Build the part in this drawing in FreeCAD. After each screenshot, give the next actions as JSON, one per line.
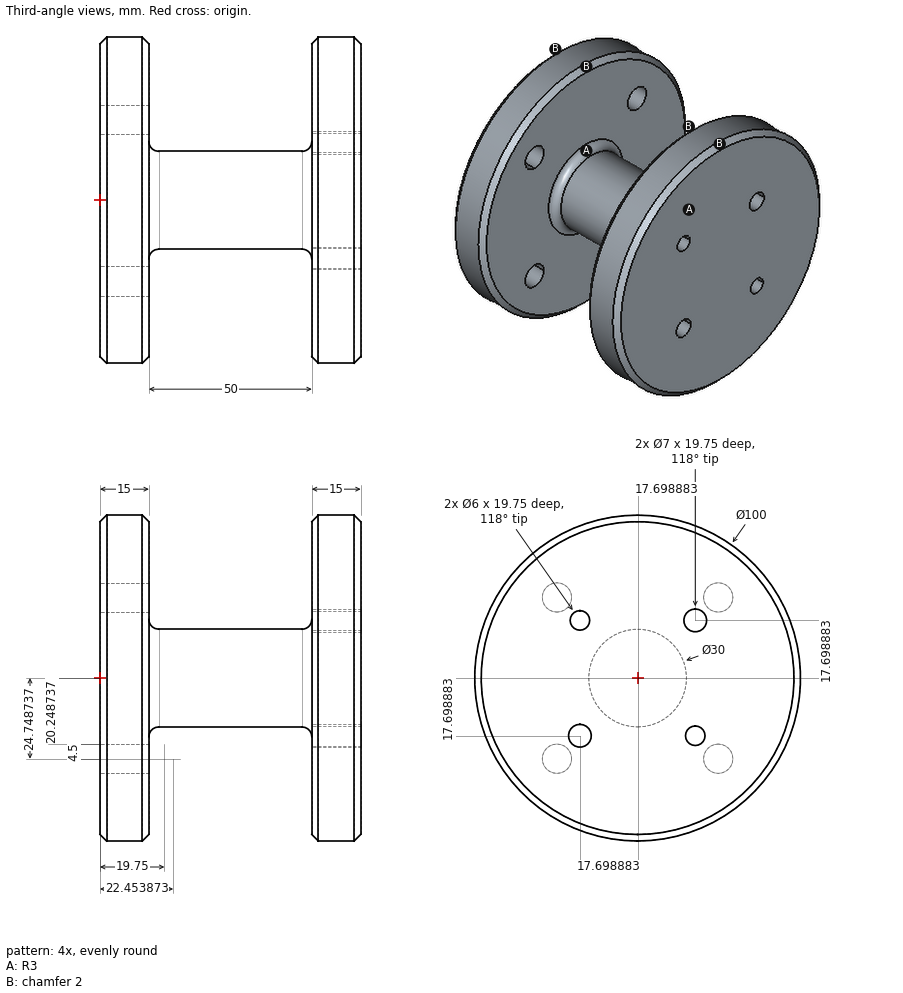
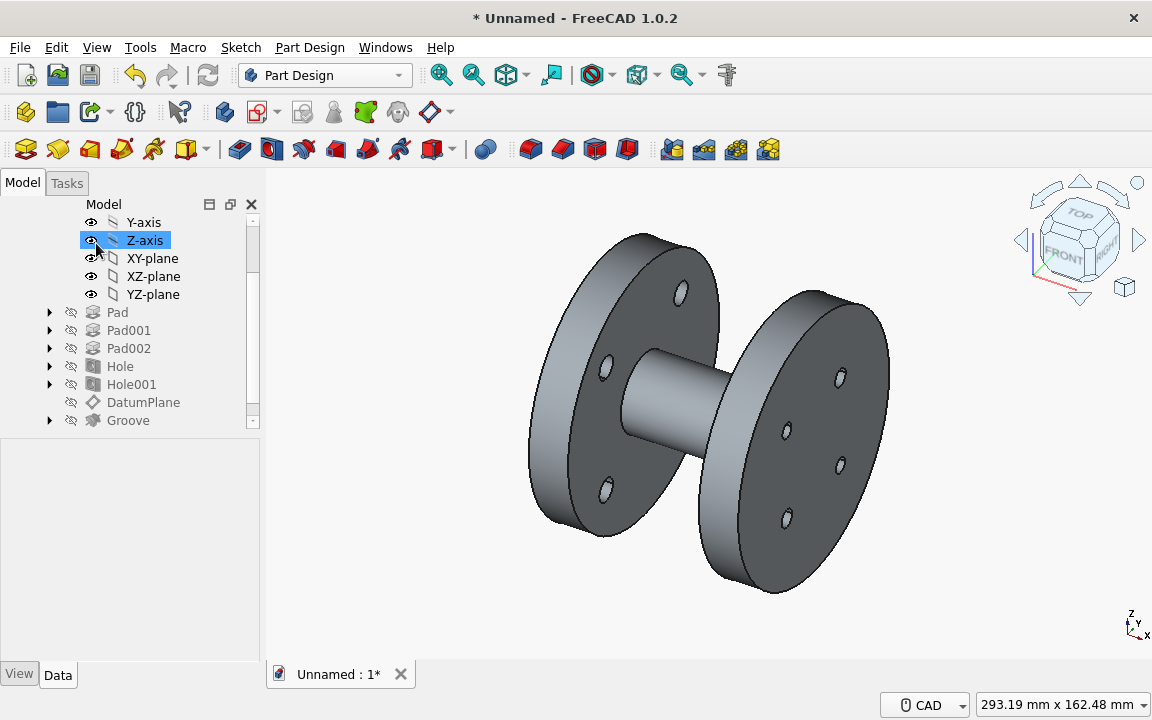
{"action": "key", "text": "0"}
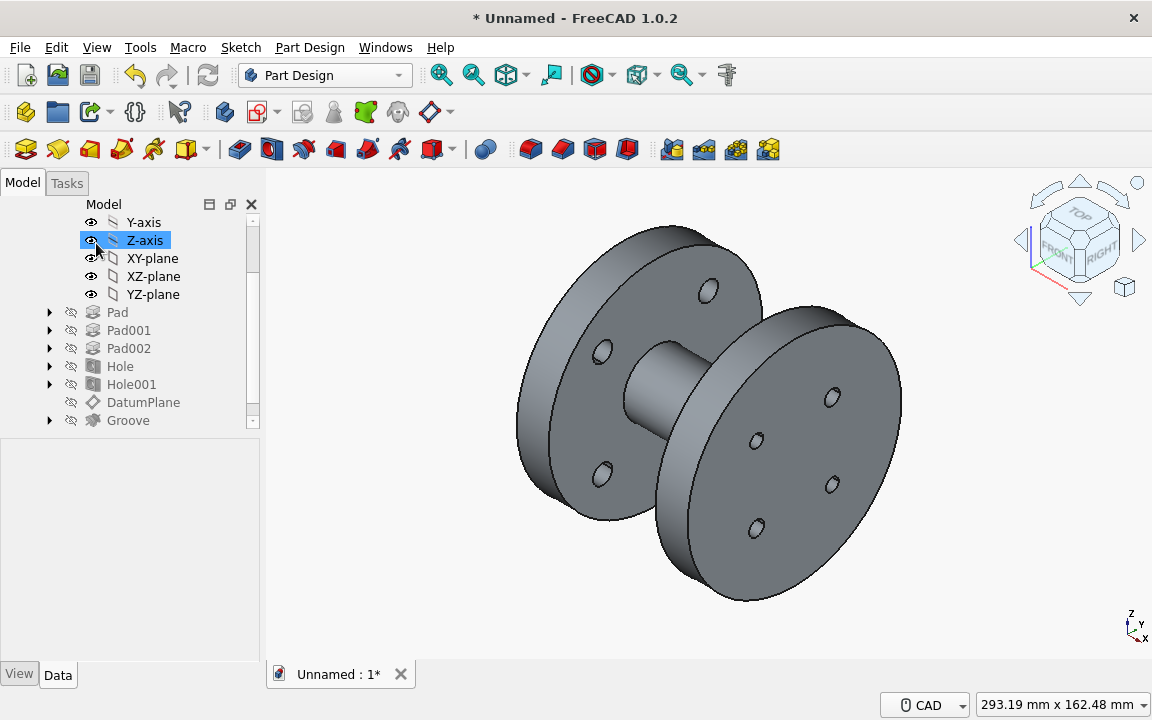
{"action": "key", "text": "2"}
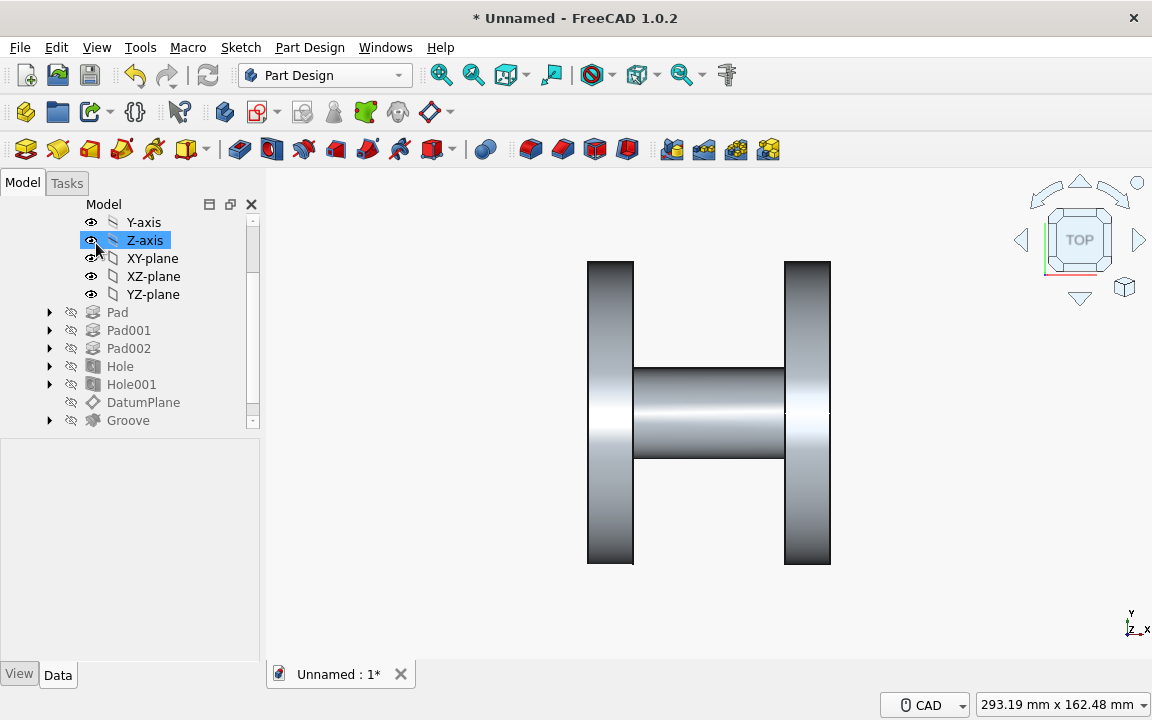
{"action": "key", "text": "1"}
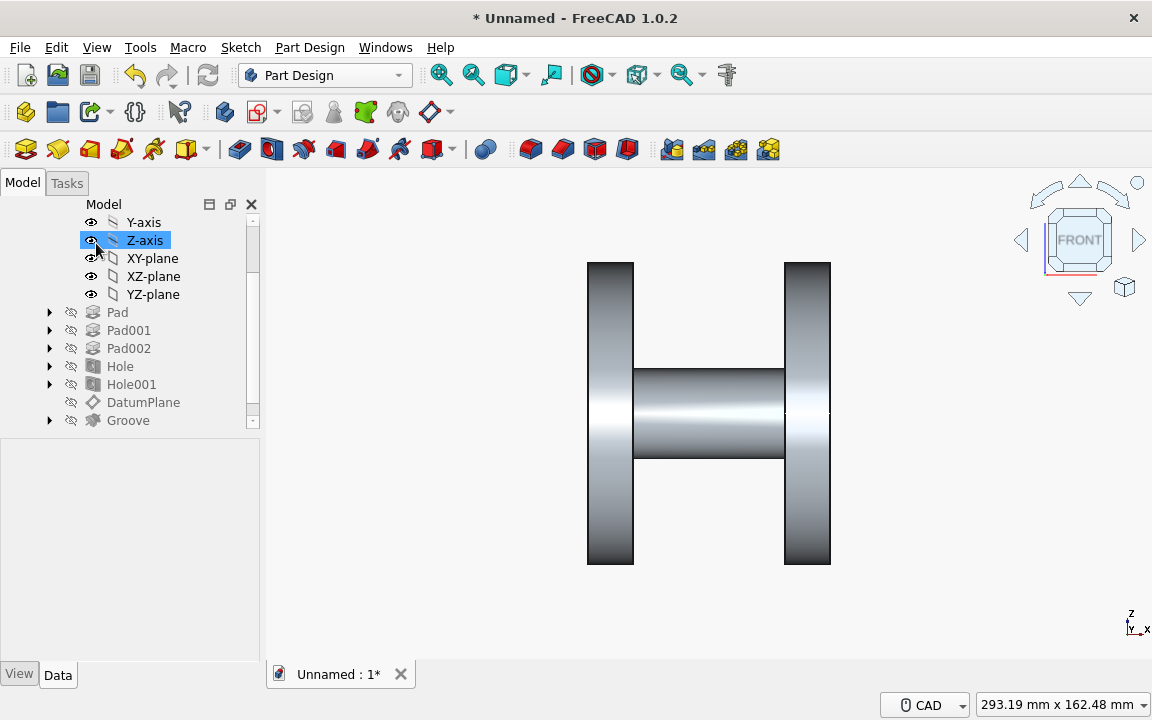
{"action": "key", "text": "3"}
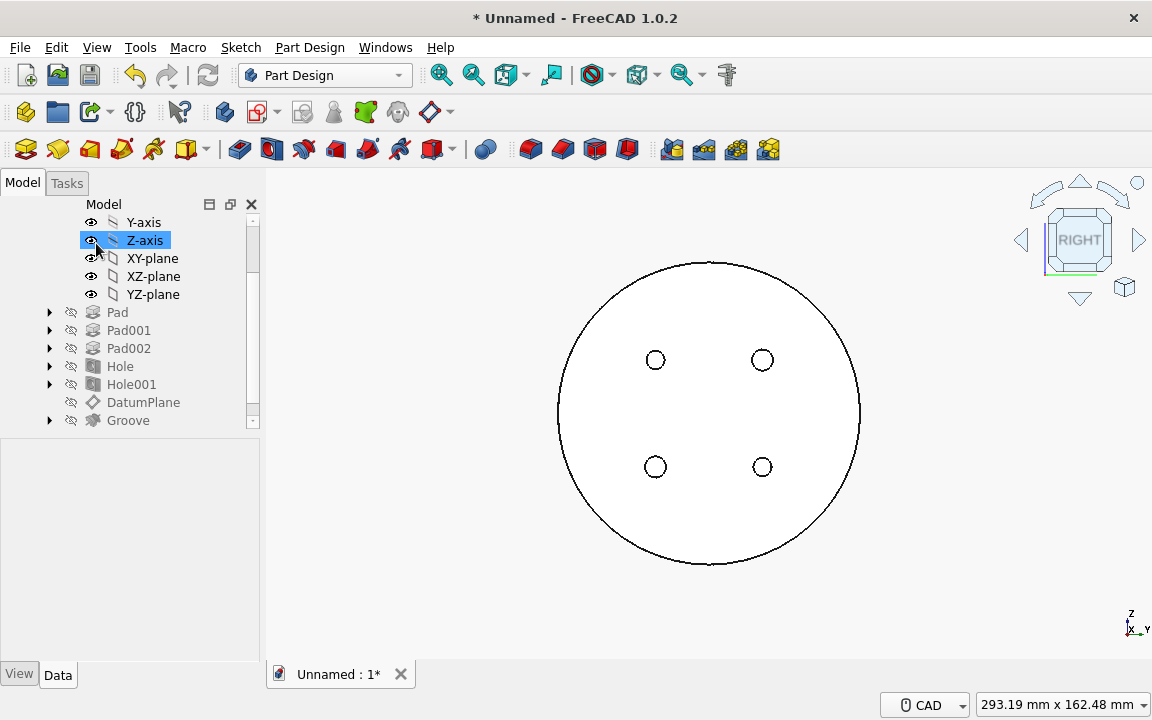
{"action": "key", "text": "5"}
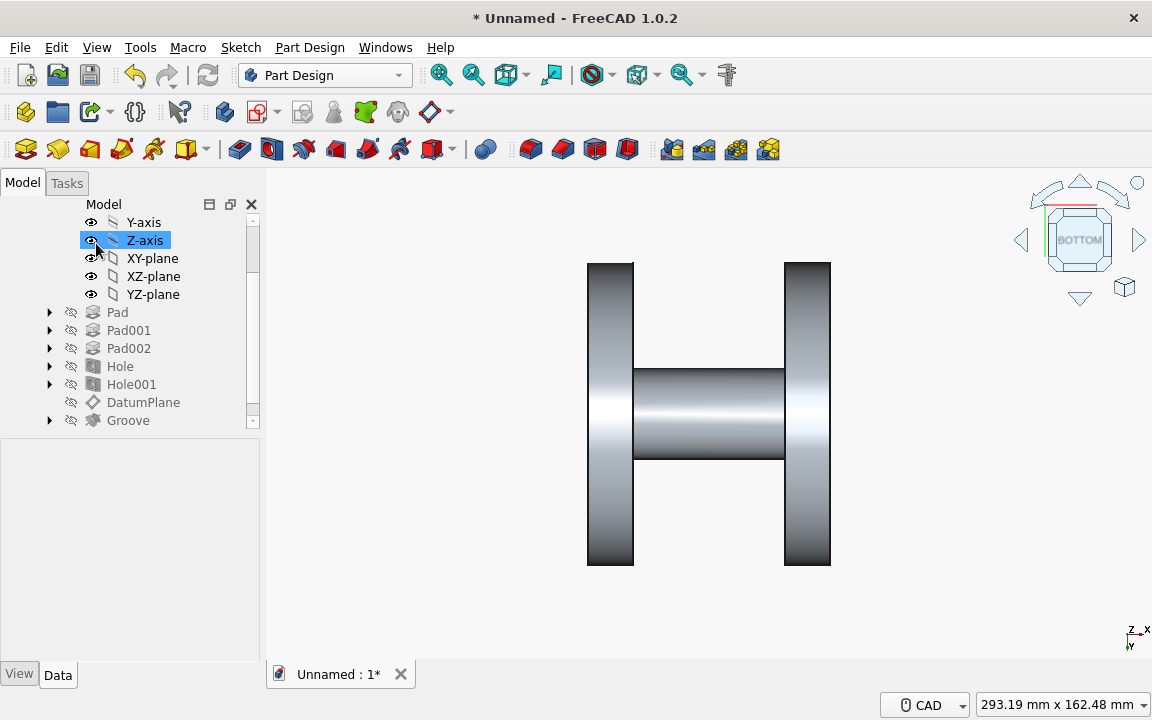
{"action": "key", "text": "4"}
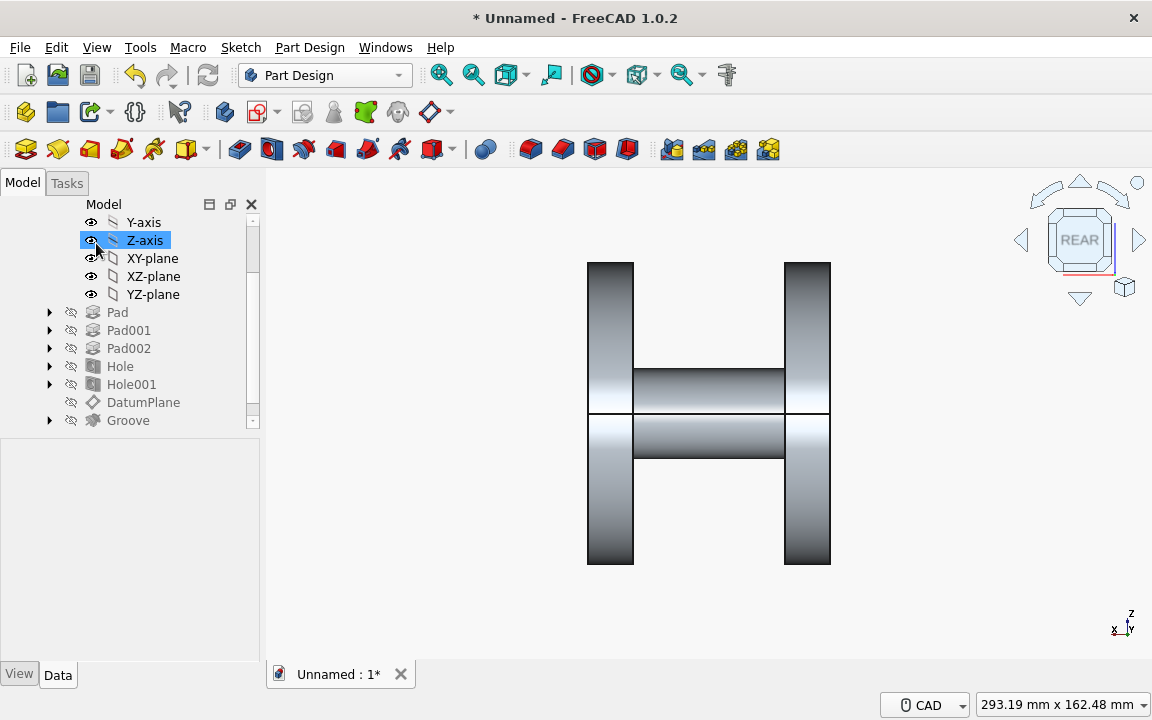
{"action": "key", "text": "6"}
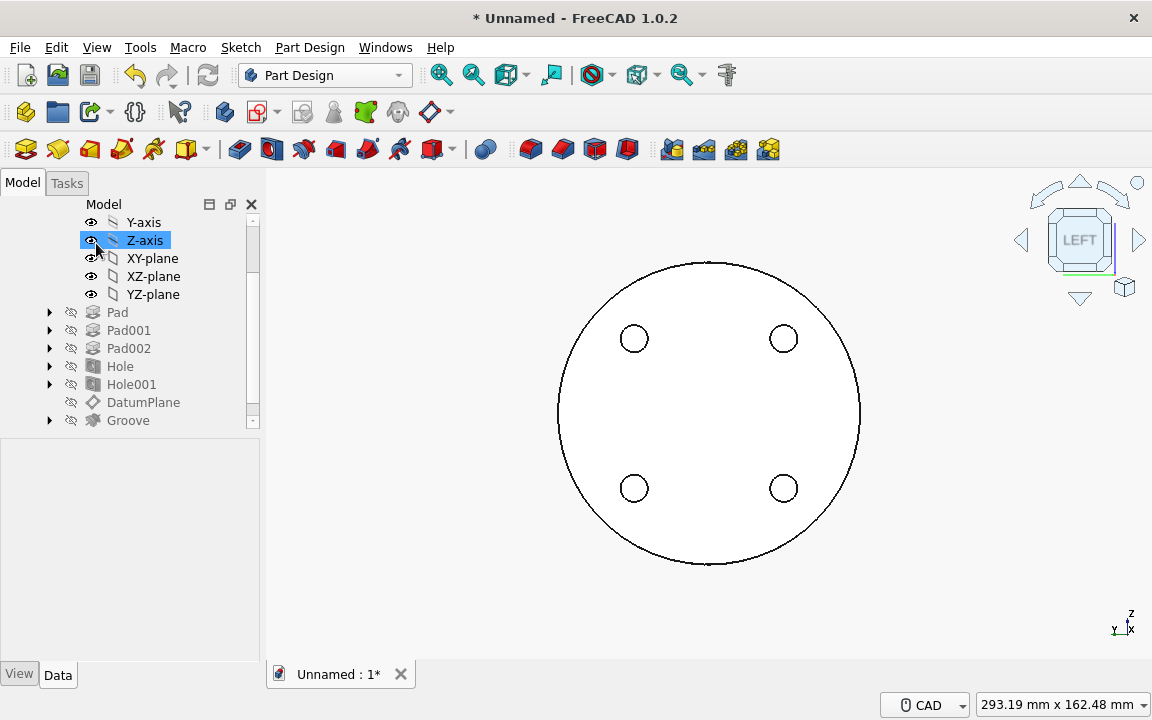
{"action": "key", "text": "v 3"}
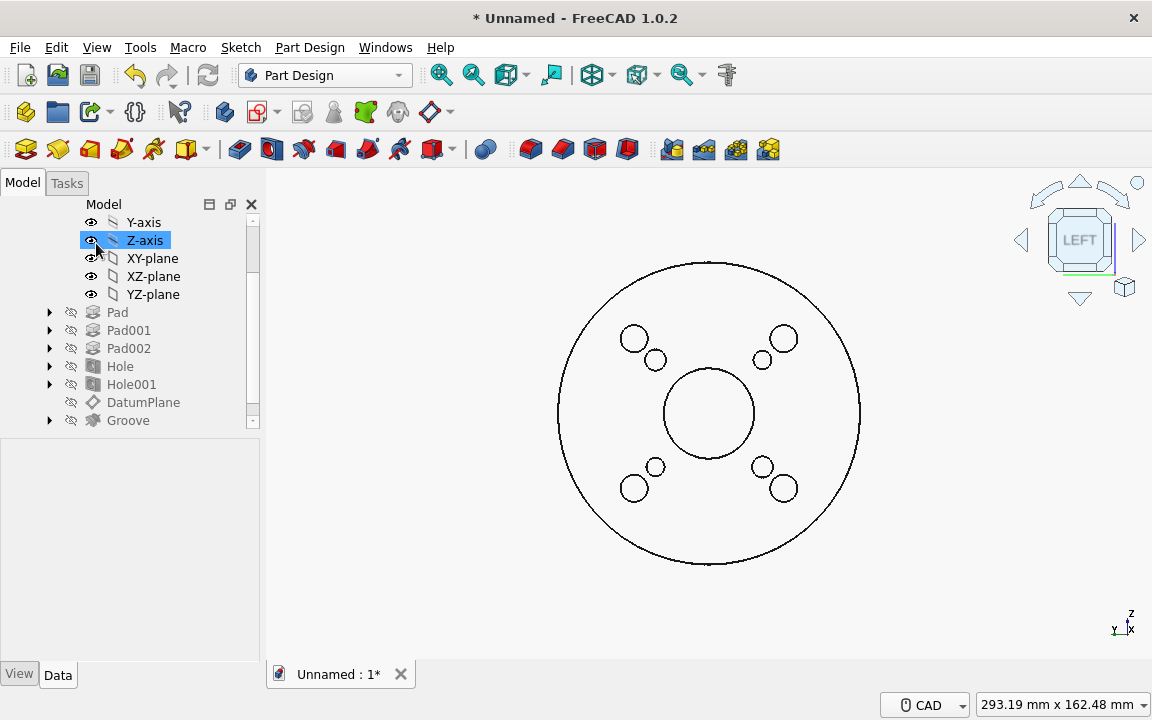
{"action": "key", "text": "0"}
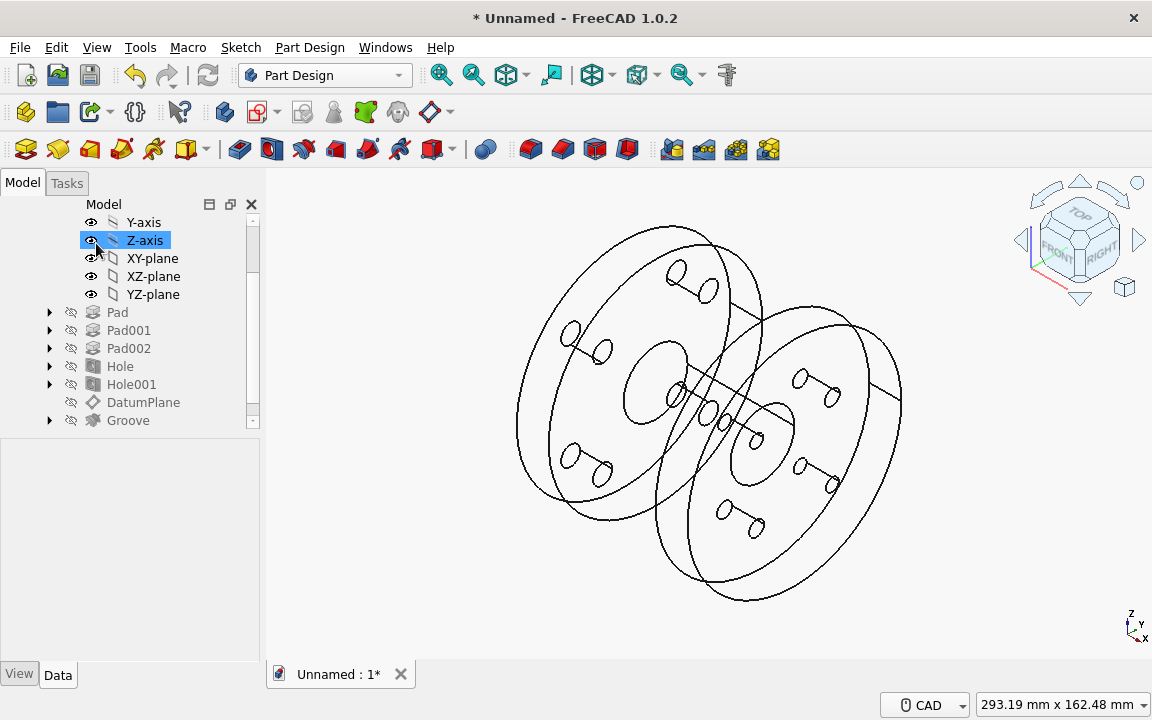
{"action": "left_click", "coordinate": [624, 400]}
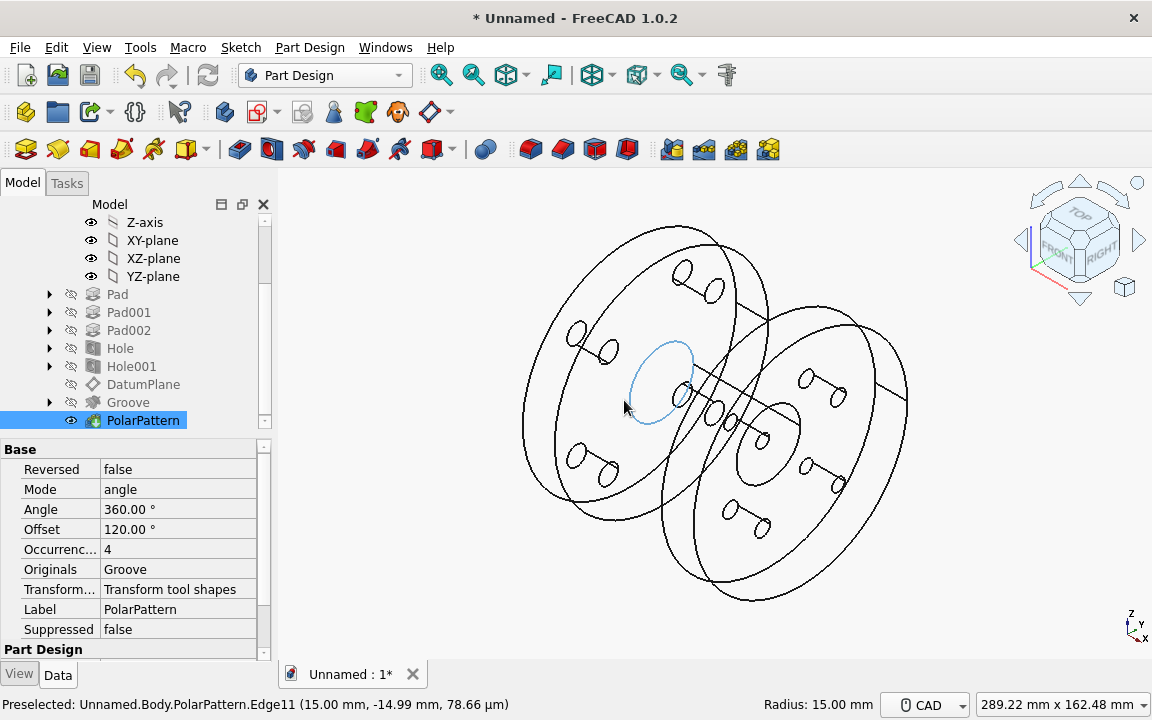
{"action": "left_click", "coordinate": [736, 462], "text": "ctrl"}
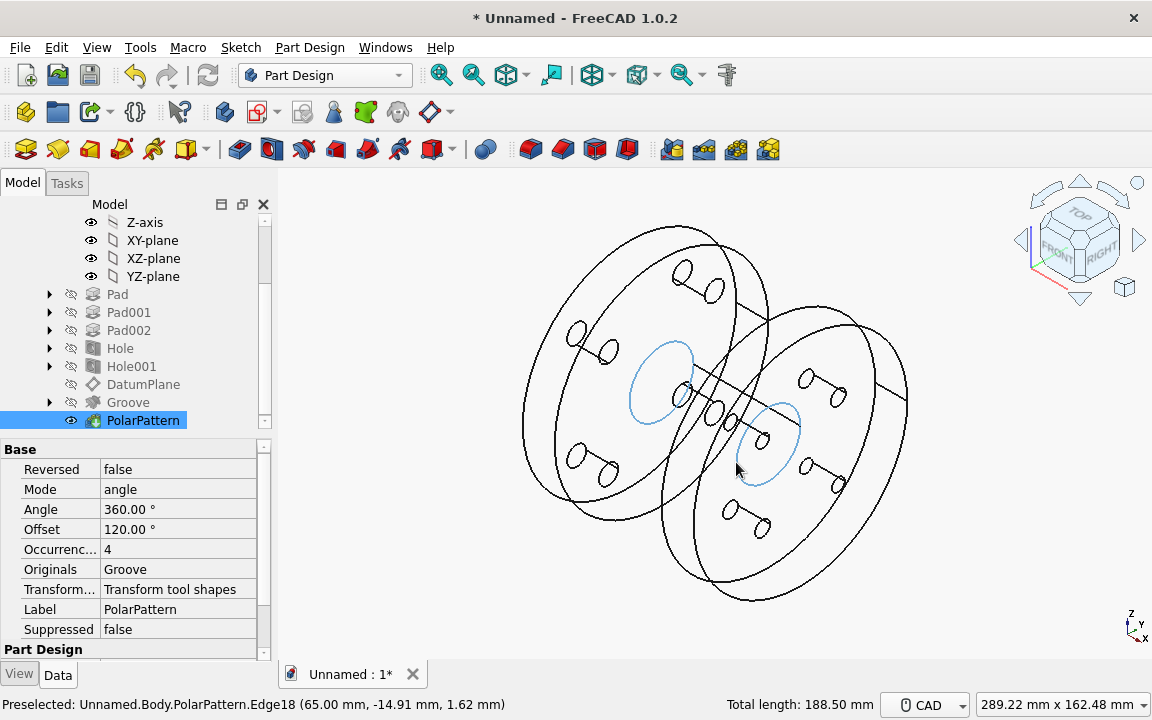
{"action": "key", "text": "v 1"}